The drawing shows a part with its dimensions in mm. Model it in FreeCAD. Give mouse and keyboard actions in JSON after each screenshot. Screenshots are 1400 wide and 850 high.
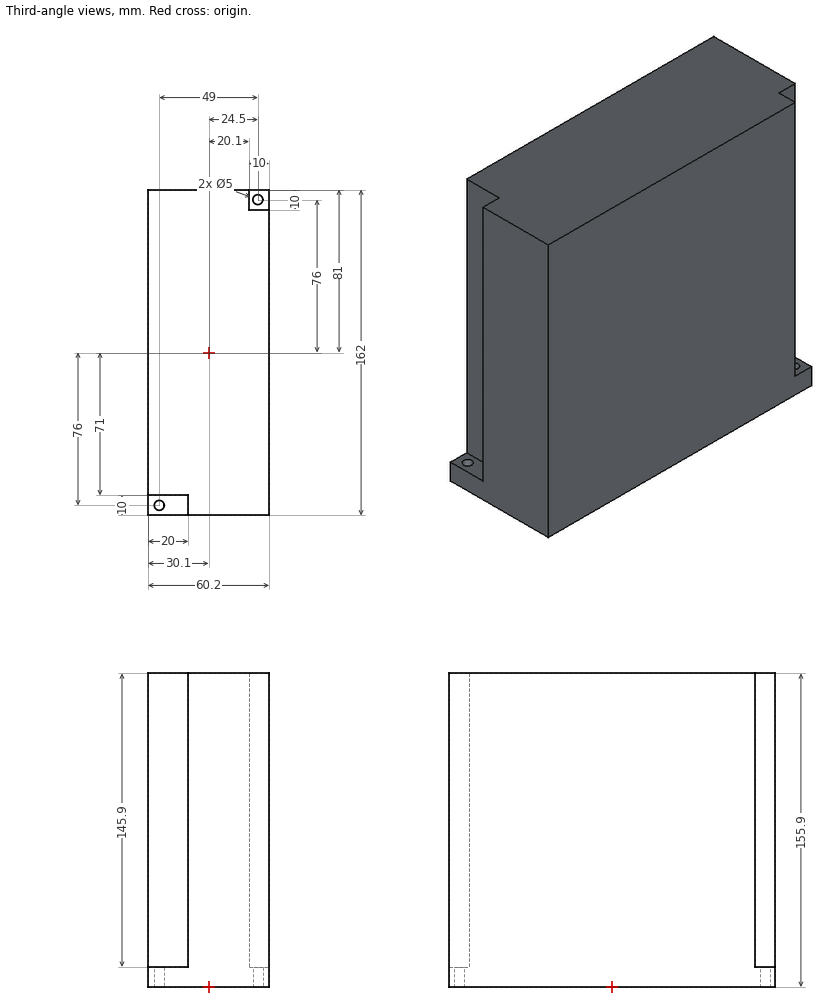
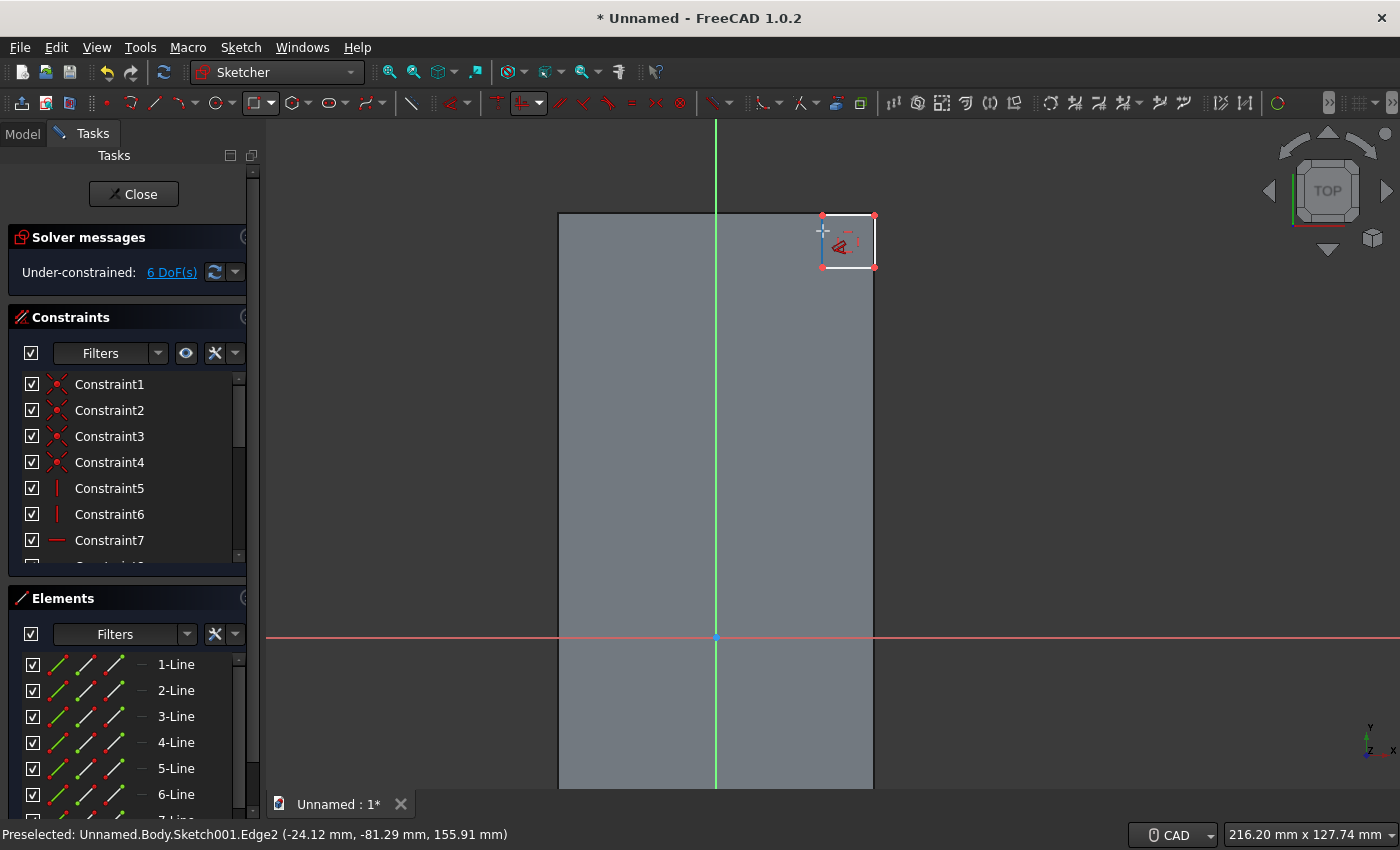
{"action": "left_click", "coordinate": [822, 231]}
{"action": "left_click", "coordinate": [856, 241]}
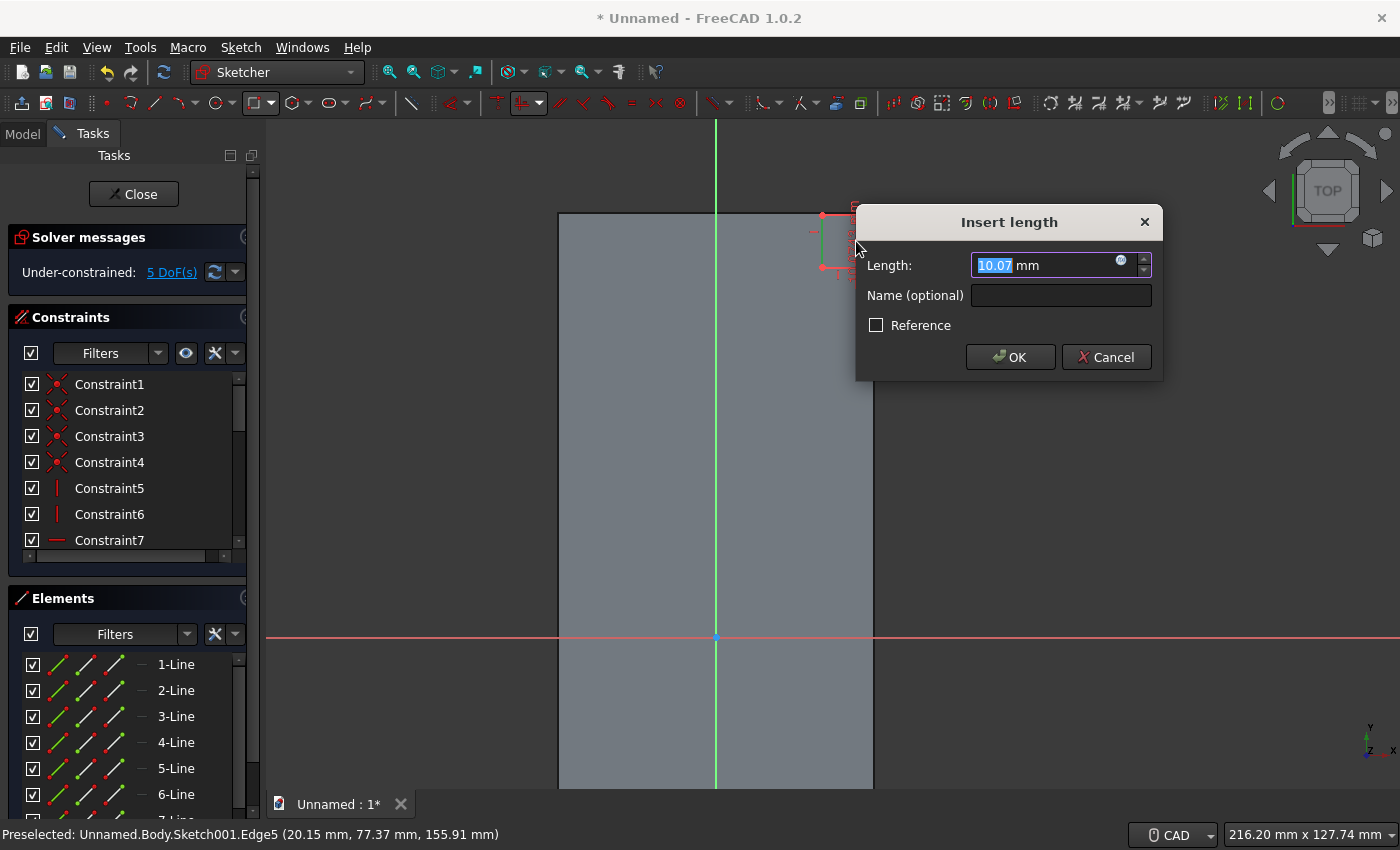
{"action": "type", "text": "10"}
{"action": "key", "text": "Return"}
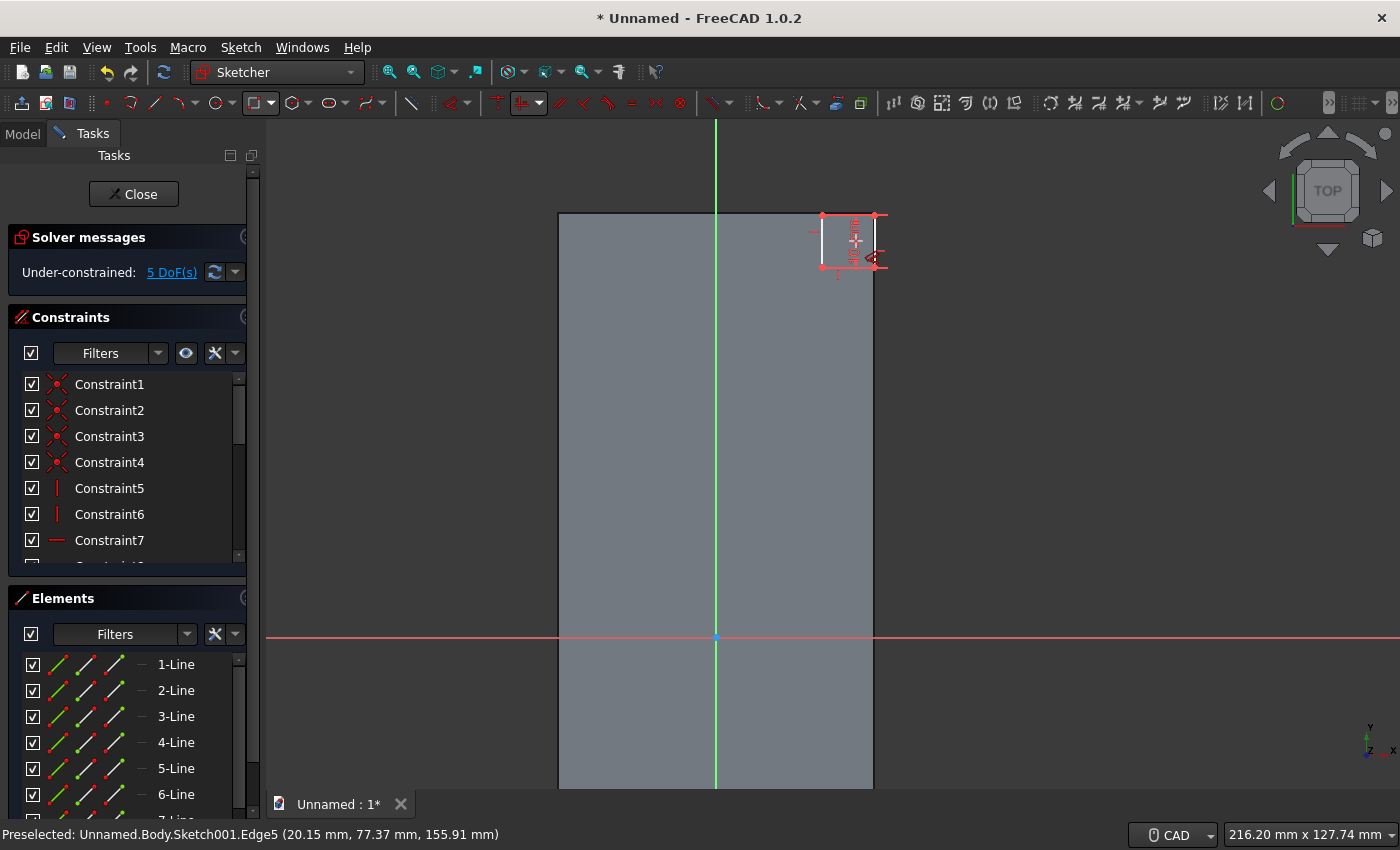
{"action": "left_click", "coordinate": [838, 268]}
{"action": "left_click", "coordinate": [848, 302]}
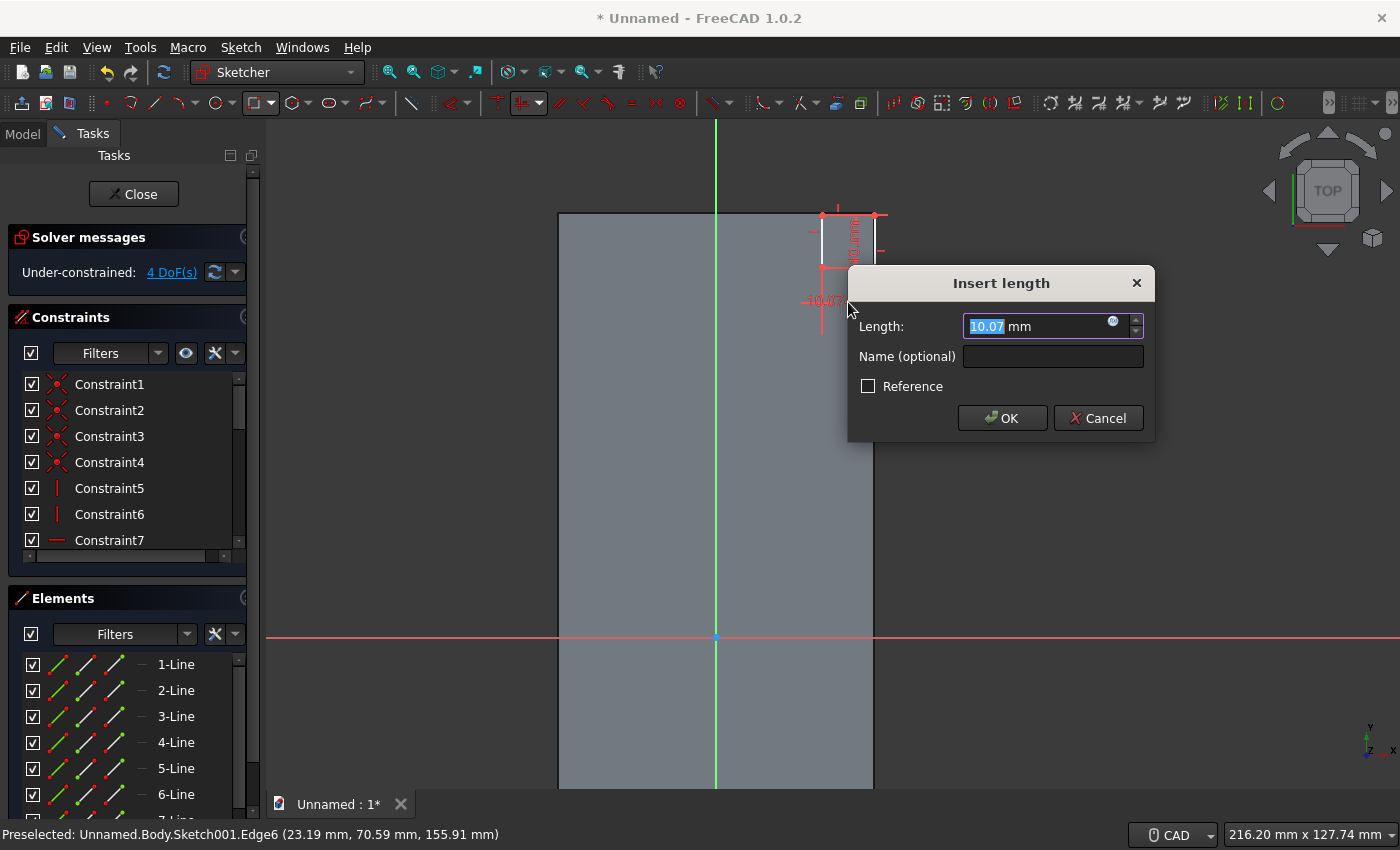
{"action": "type", "text": "10"}
{"action": "key", "text": "Return"}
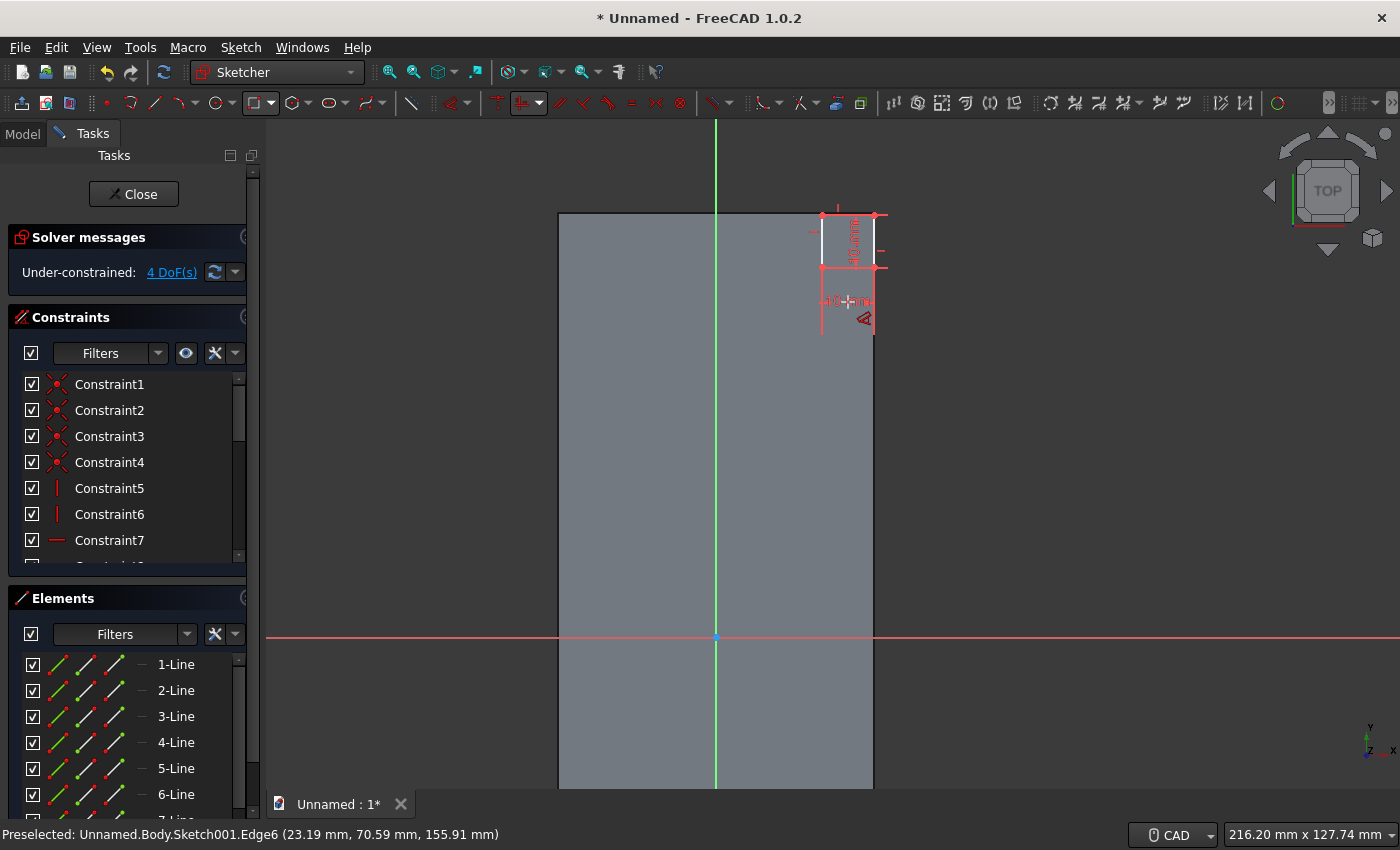
{"action": "scroll", "coordinate": [823, 230], "scroll_direction": "down", "scroll_amount": 3}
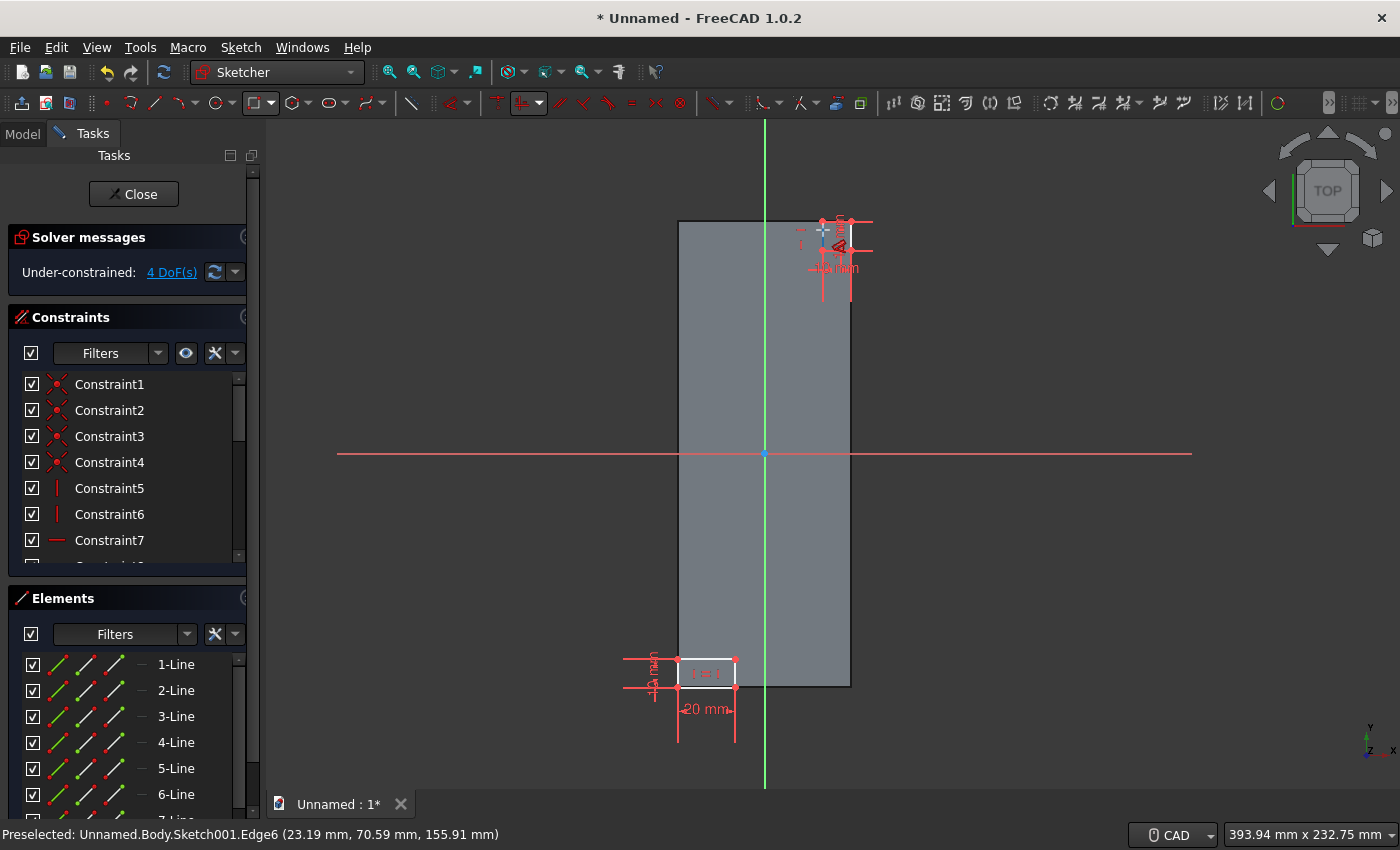
{"action": "left_click", "coordinate": [678, 659]}
{"action": "left_click", "coordinate": [644, 556]}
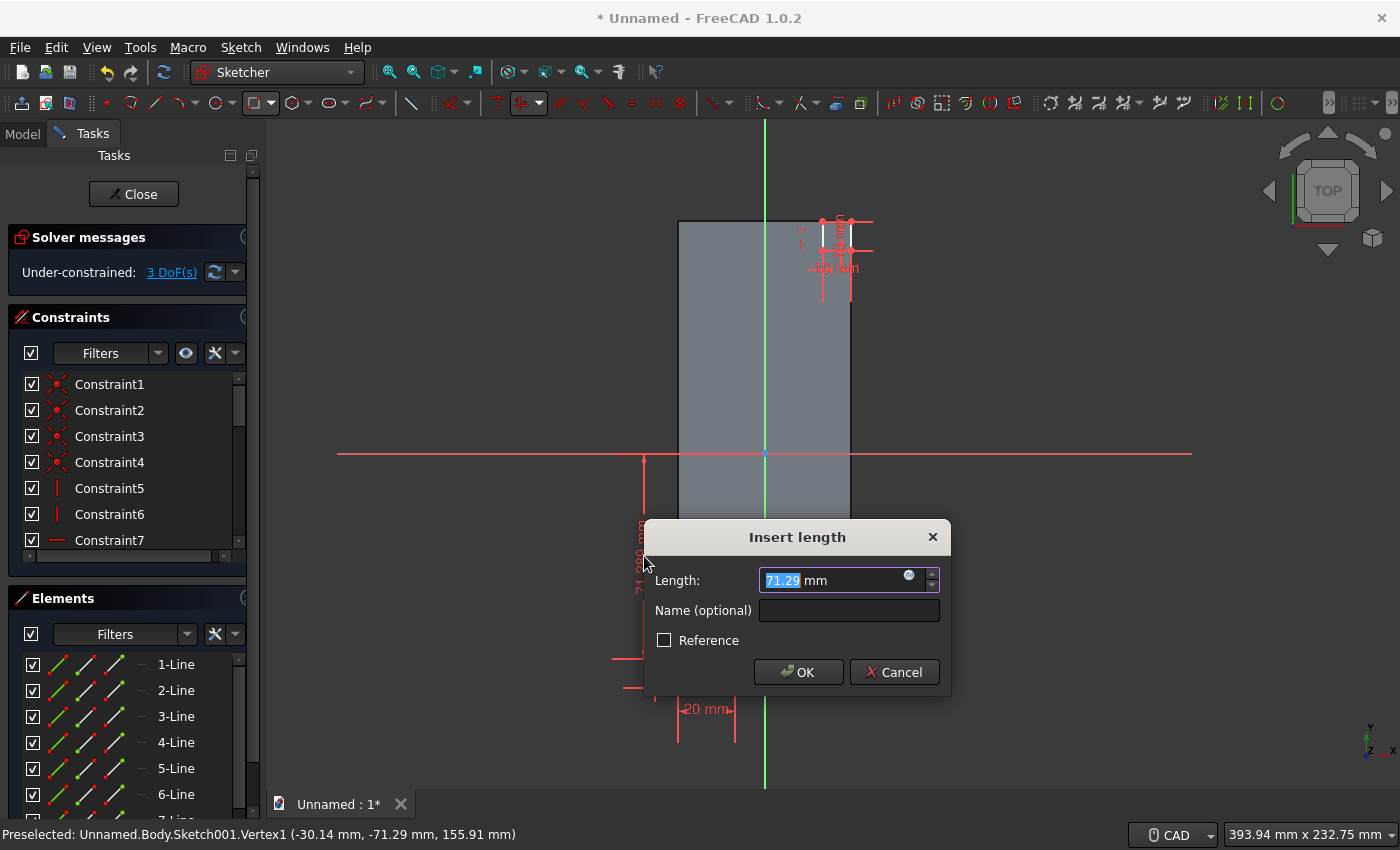
{"action": "type", "text": "71"}
{"action": "key", "text": "Return"}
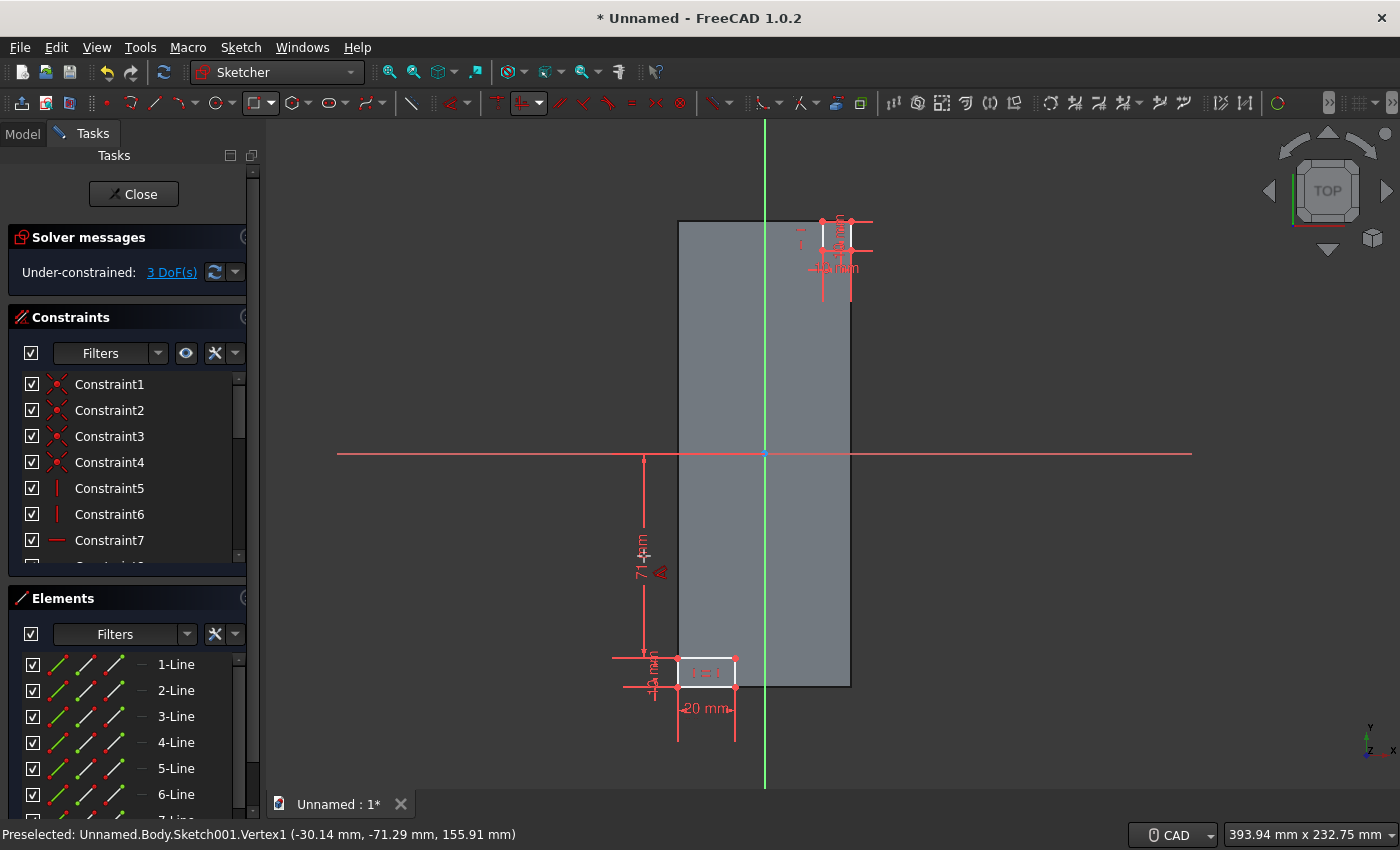
{"action": "left_click", "coordinate": [823, 222]}
{"action": "left_click", "coordinate": [857, 338]}